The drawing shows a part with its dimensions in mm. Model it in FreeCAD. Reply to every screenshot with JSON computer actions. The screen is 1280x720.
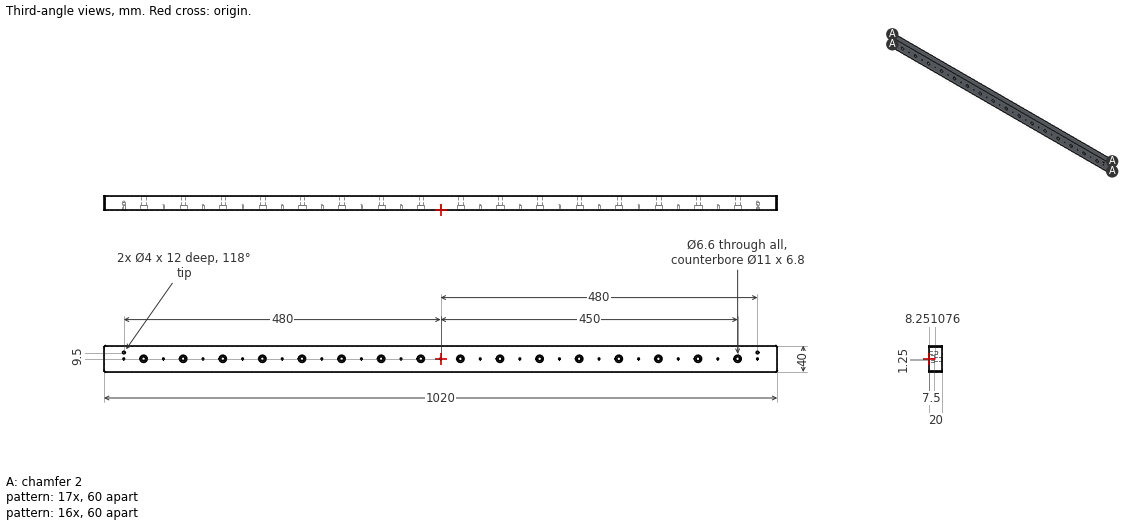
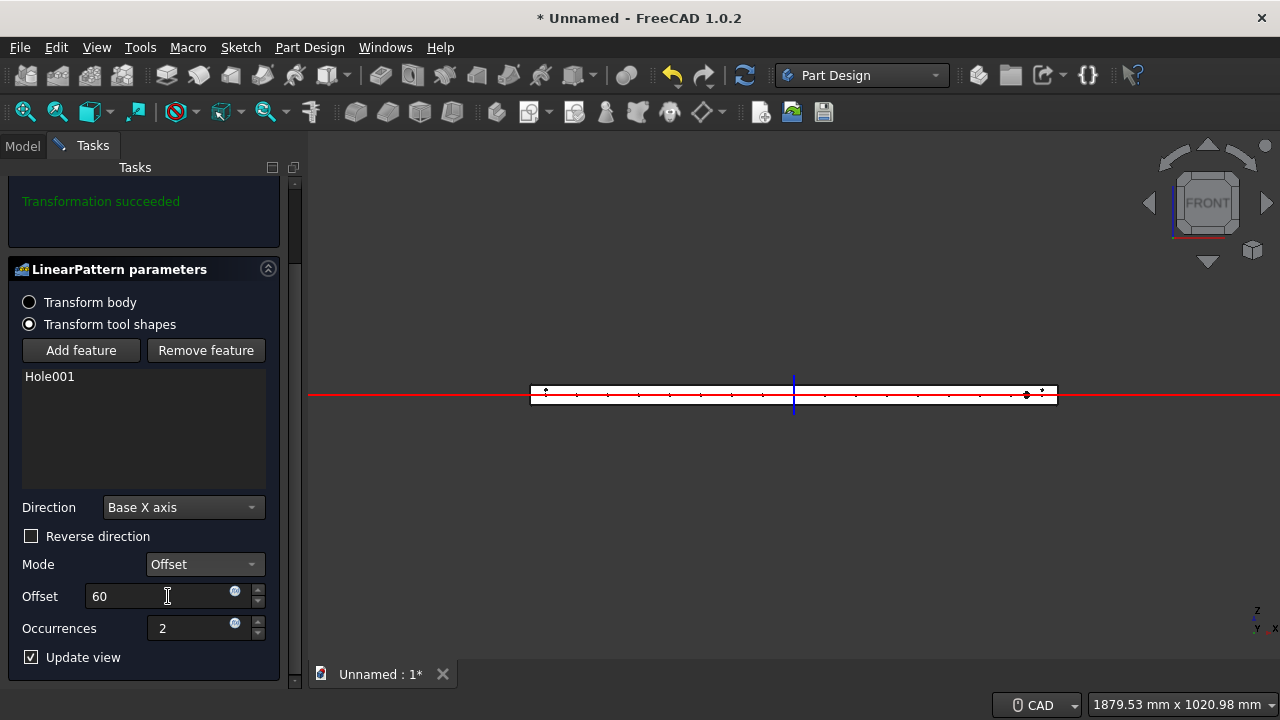
{"action": "triple_click", "coordinate": [198, 628]}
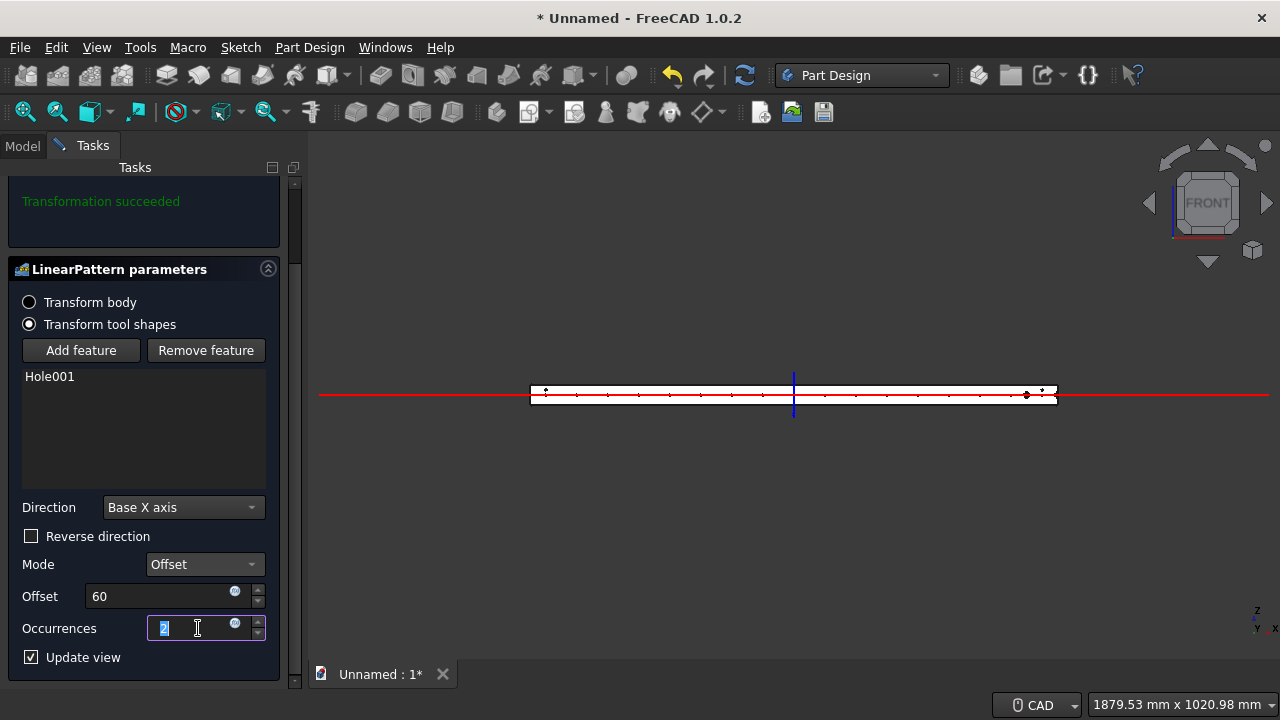
{"action": "type", "text": "16"}
{"action": "key", "text": "Tab"}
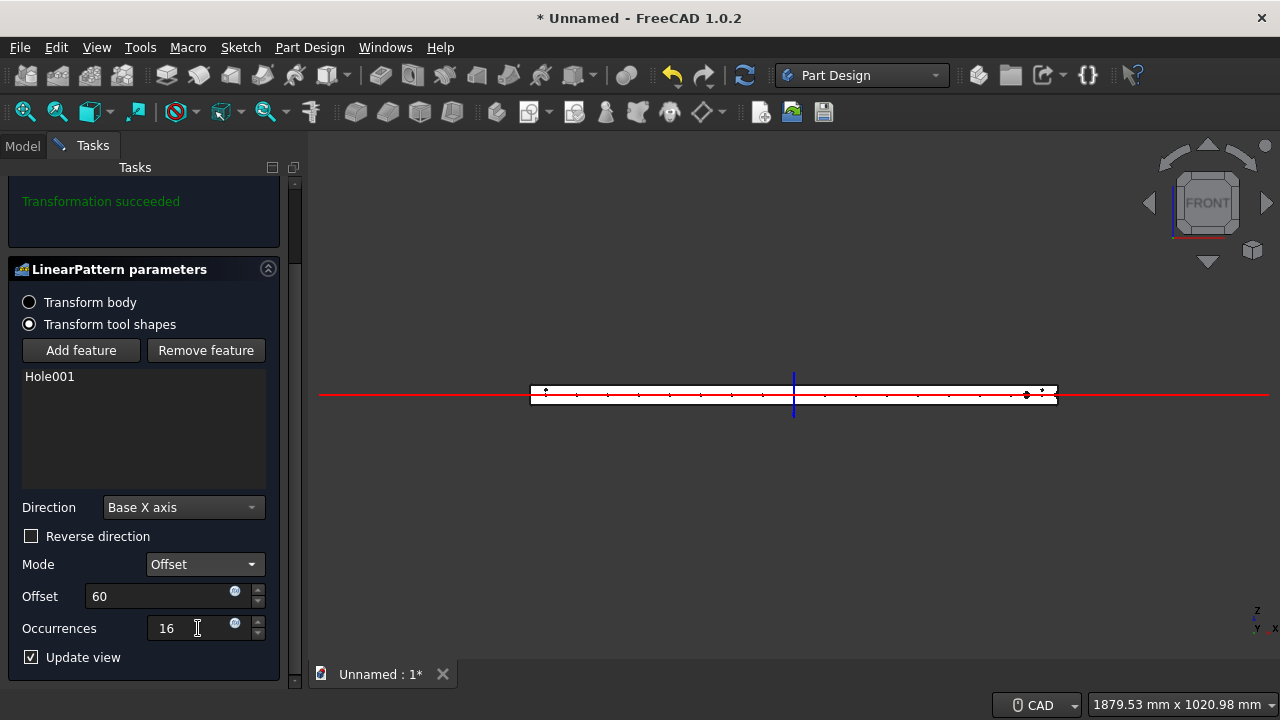
{"action": "left_click", "coordinate": [30, 536]}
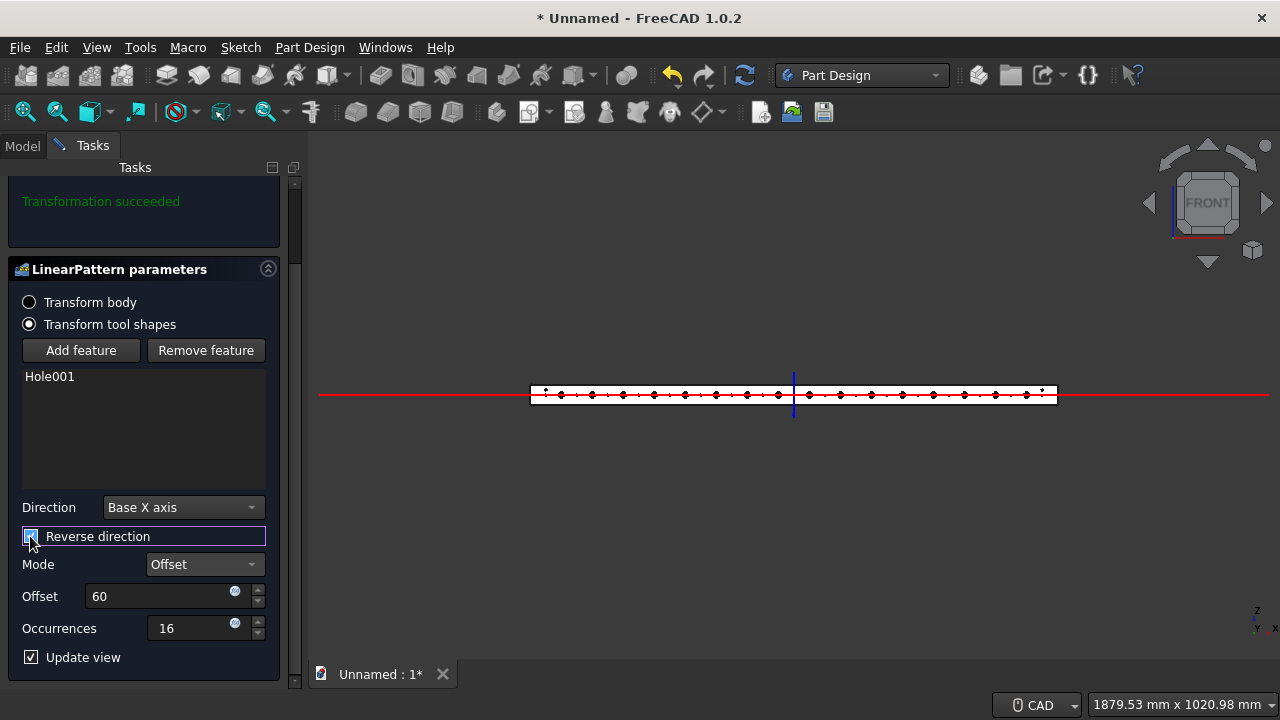
{"action": "scroll", "coordinate": [295, 432], "scroll_direction": "up", "scroll_amount": 3}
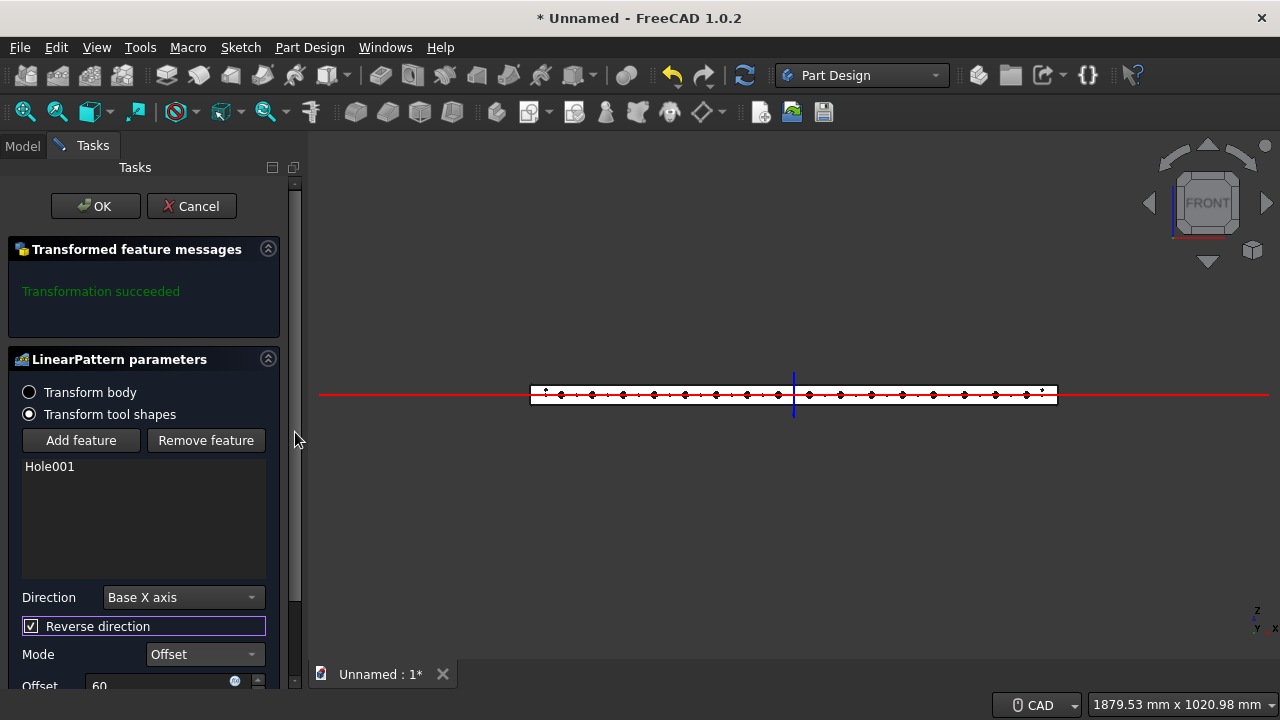
{"action": "left_click", "coordinate": [96, 206]}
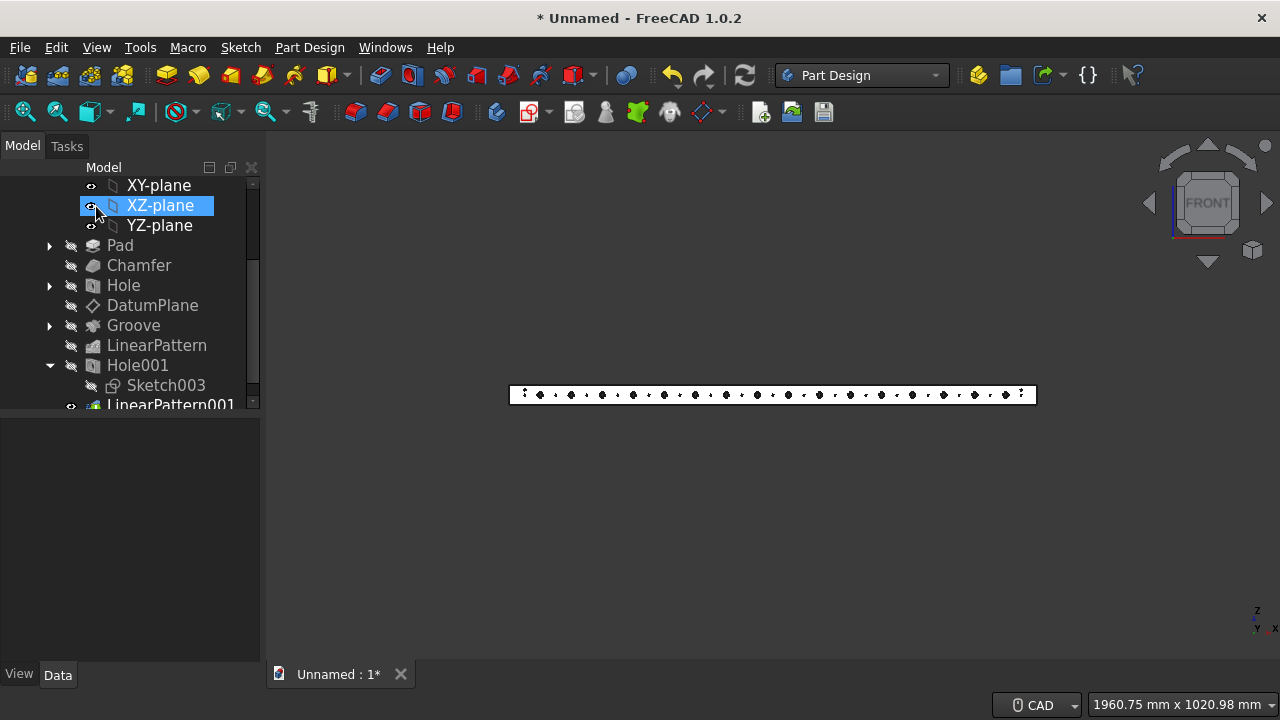
{"action": "key", "text": "0"}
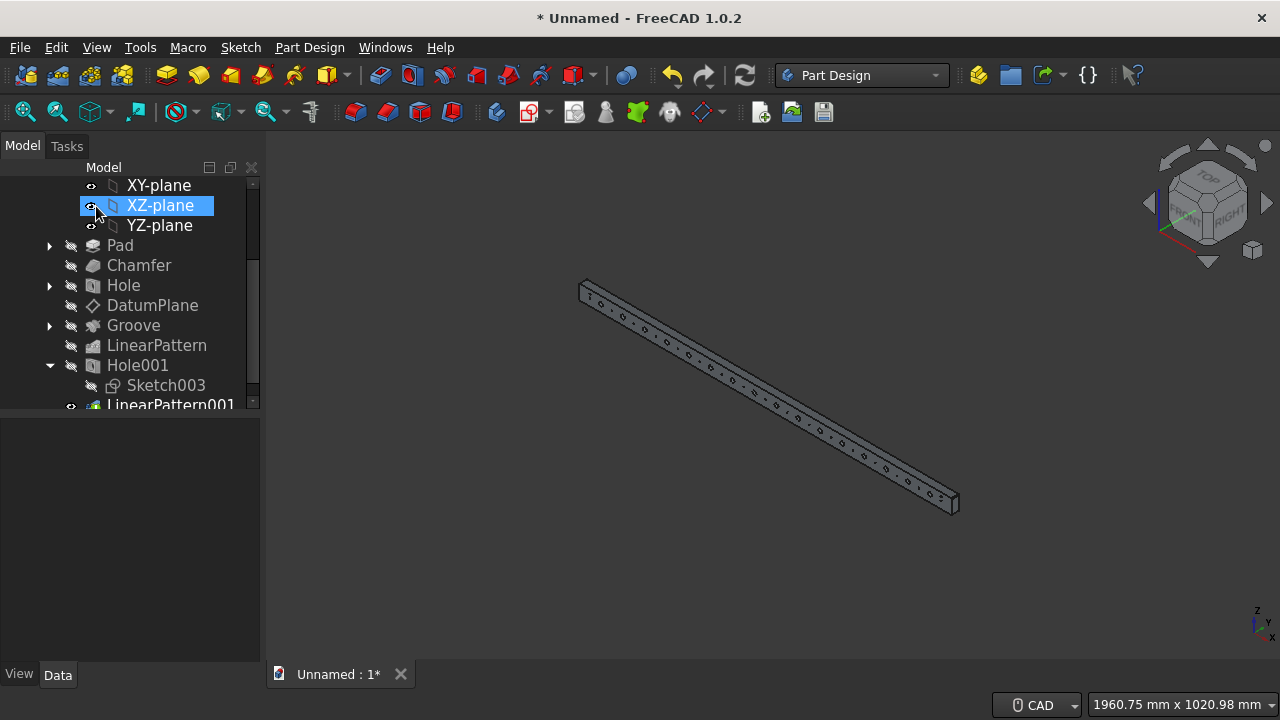
{"action": "key", "text": "v f"}